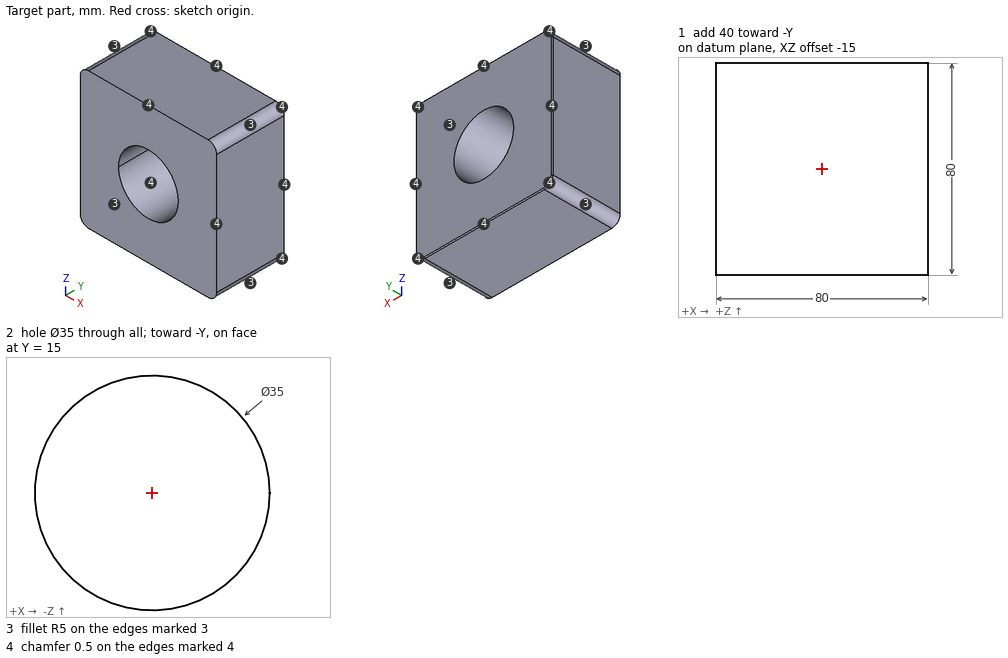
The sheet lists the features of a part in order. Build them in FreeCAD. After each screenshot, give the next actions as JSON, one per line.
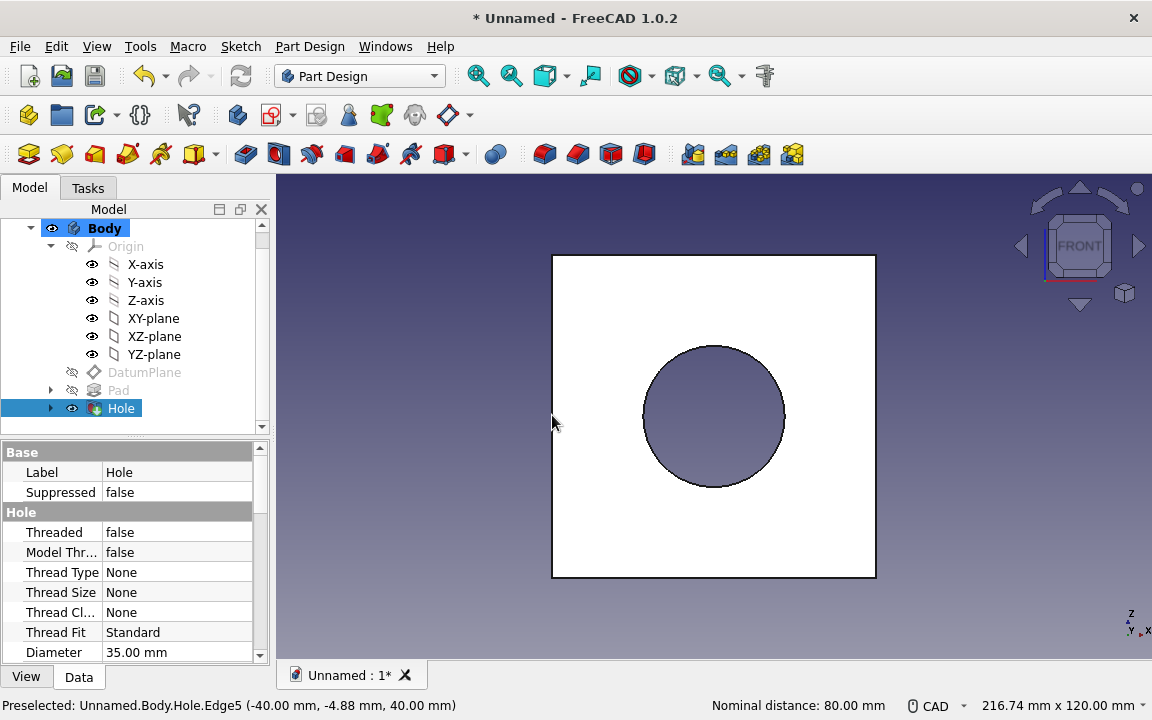
{"action": "key", "text": "3"}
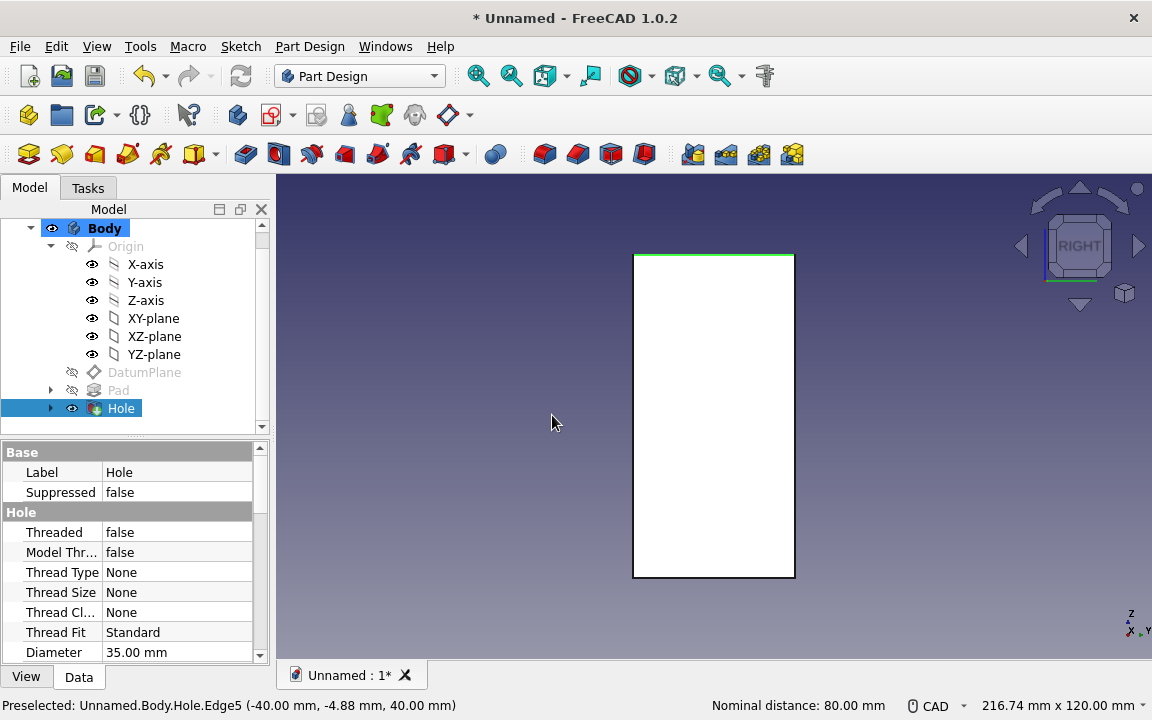
{"action": "left_click", "coordinate": [714, 577], "text": "ctrl"}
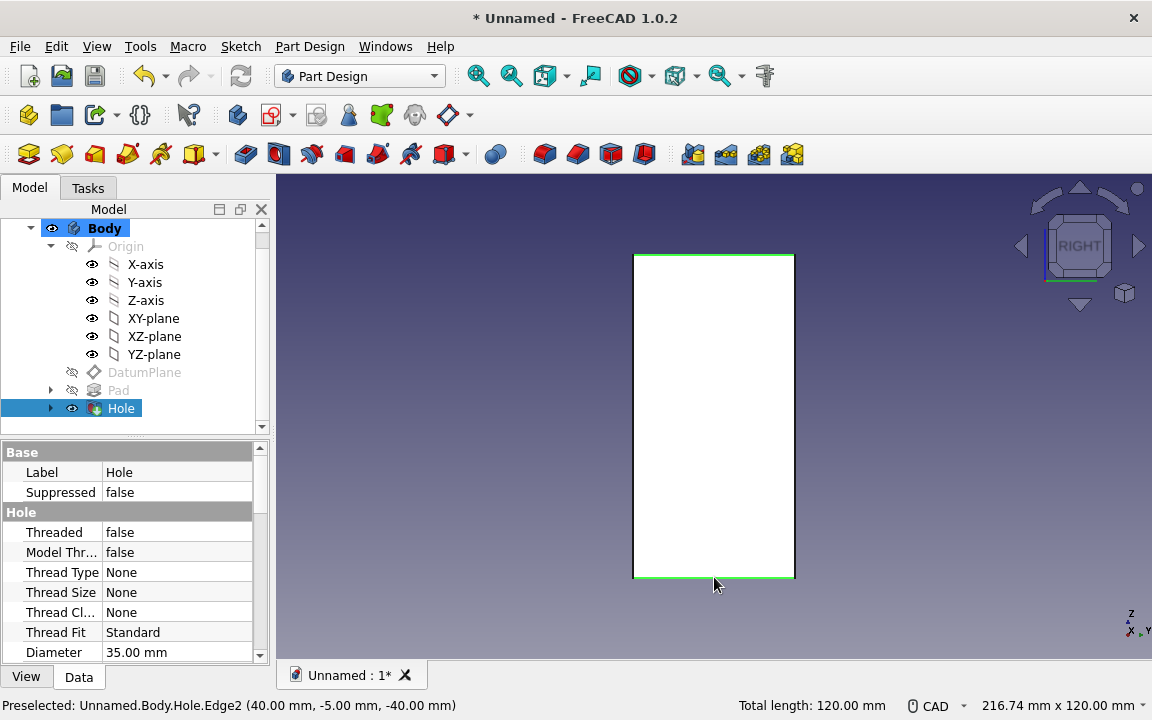
{"action": "key", "text": "5"}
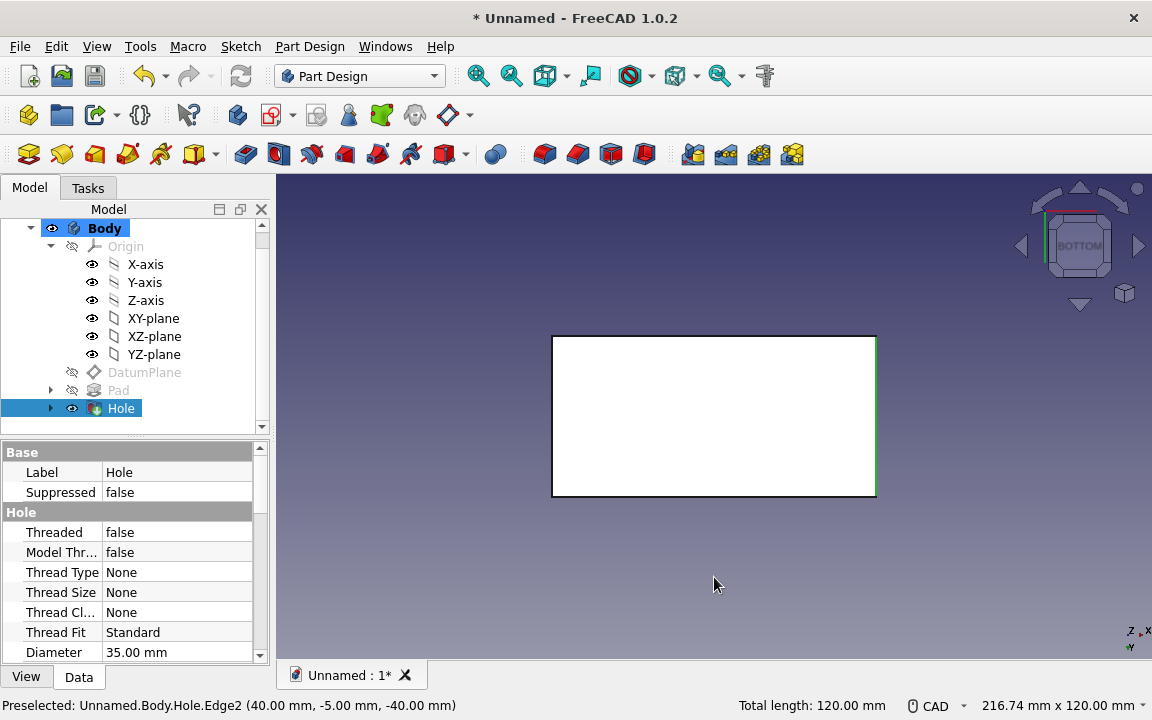
{"action": "left_click", "coordinate": [479, 76]}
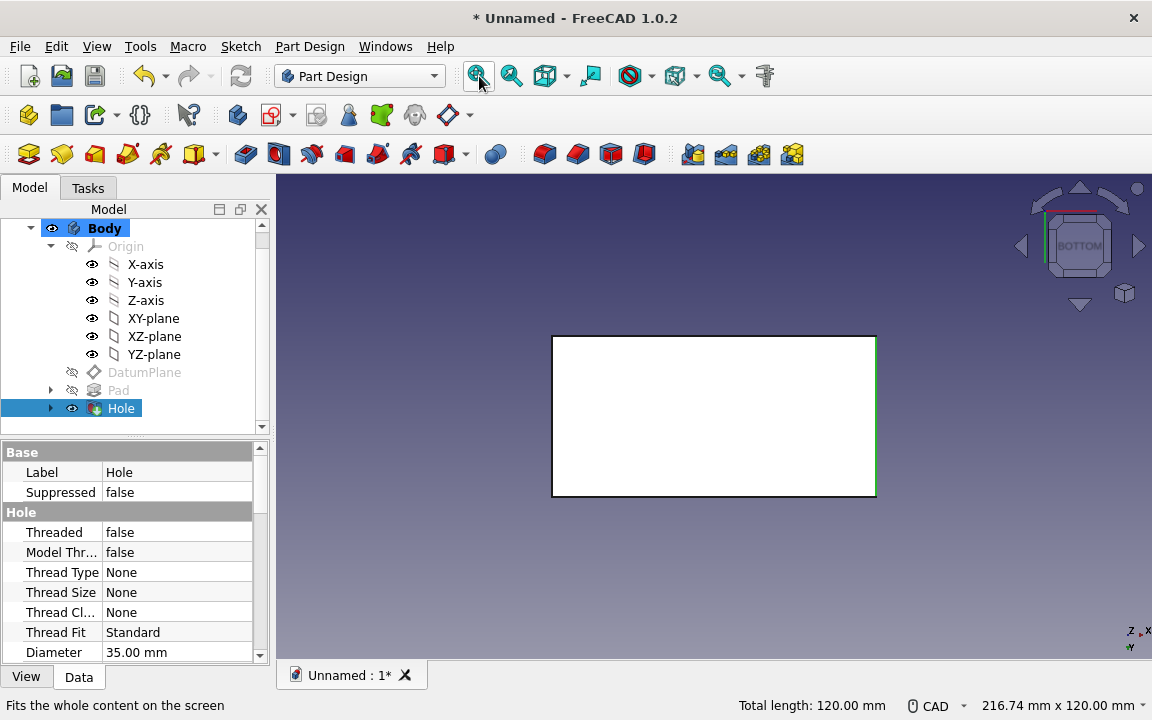
{"action": "left_click", "coordinate": [552, 415], "text": "ctrl"}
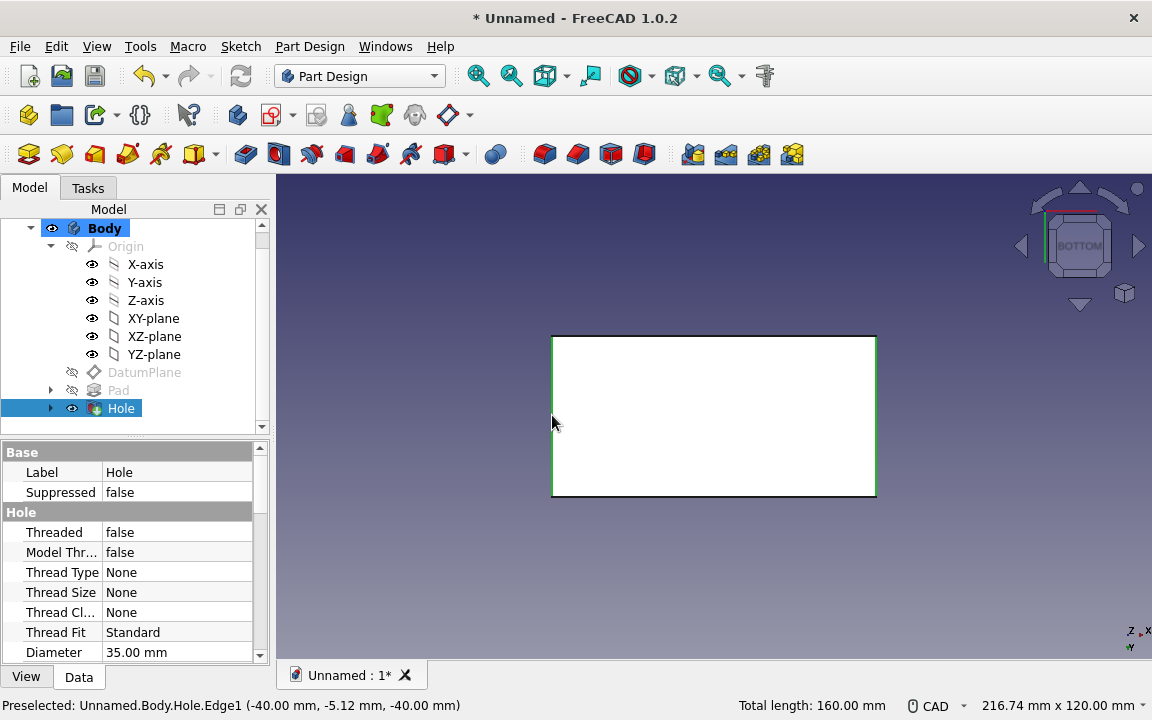
{"action": "left_click", "coordinate": [545, 154]}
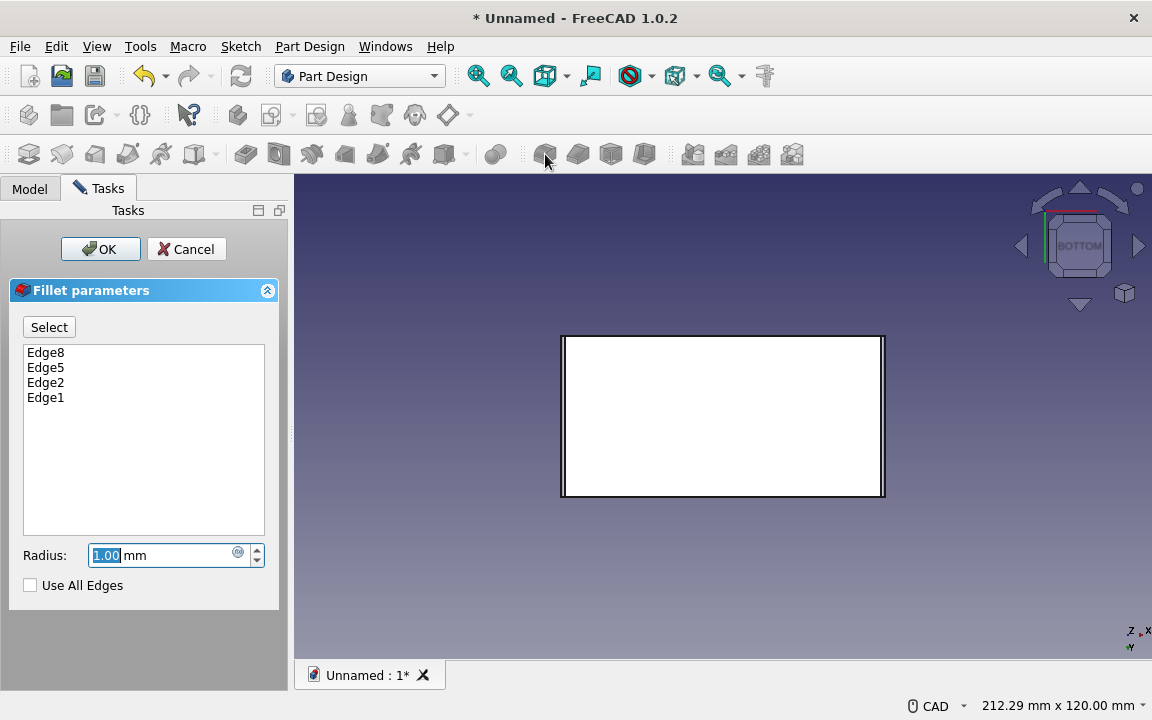
{"action": "type", "text": "5"}
{"action": "key", "text": "Tab"}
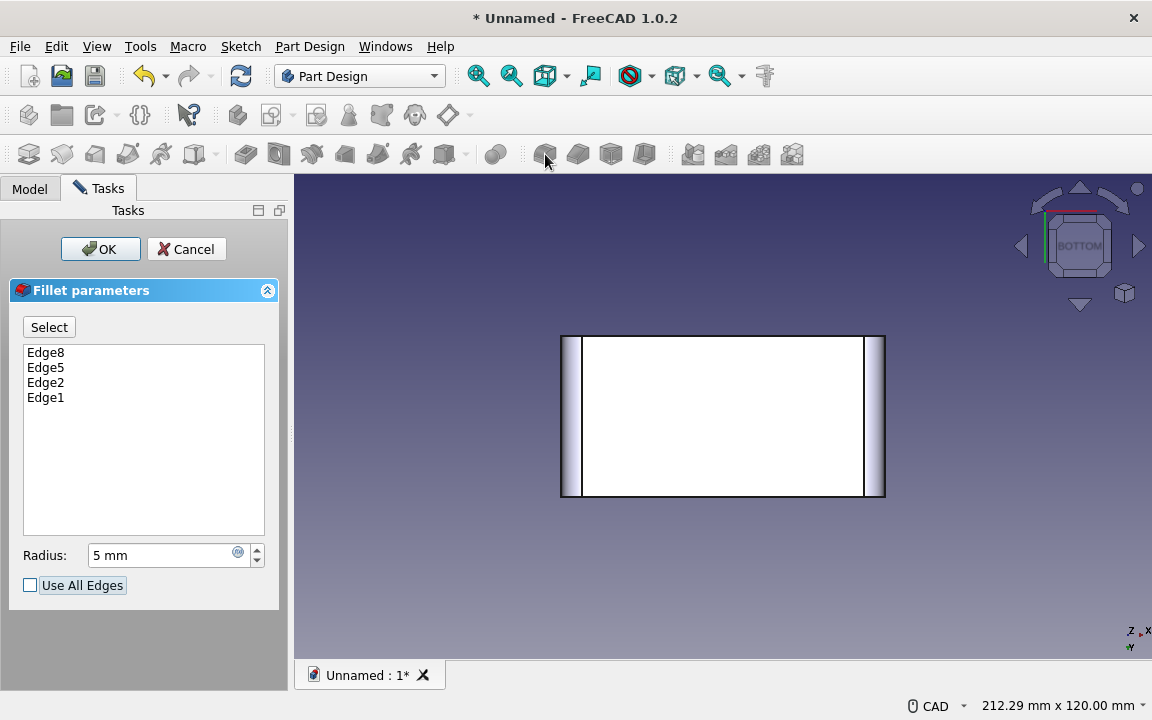
{"action": "left_click", "coordinate": [101, 249]}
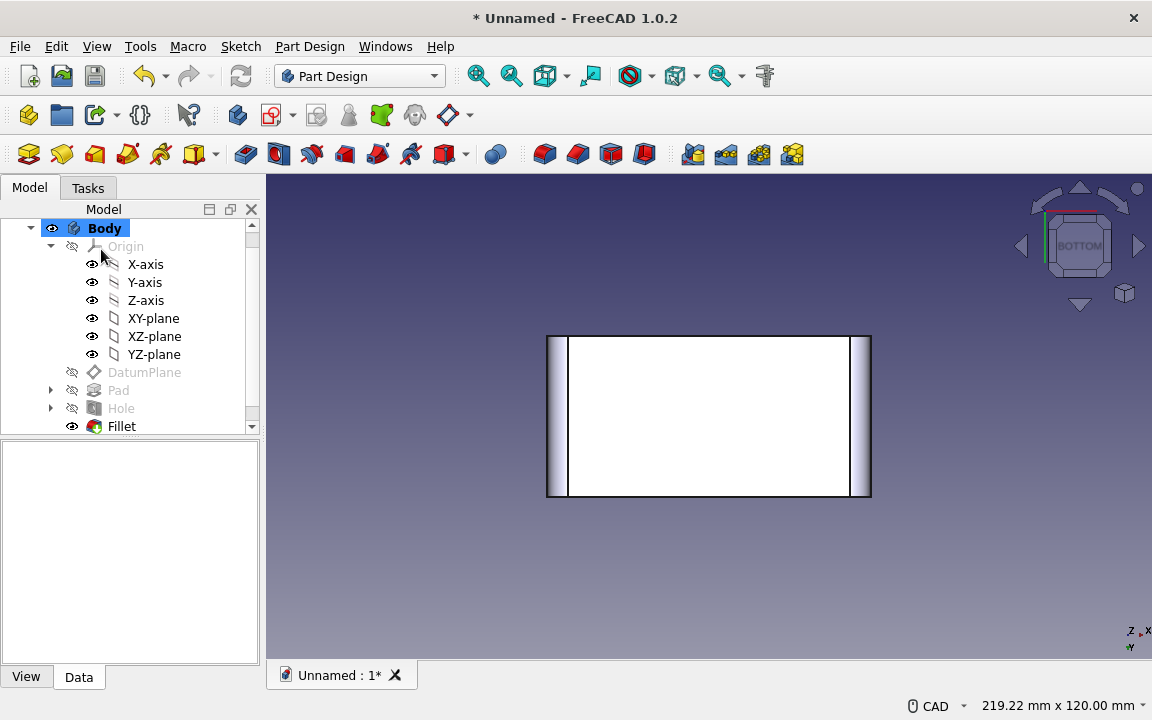
{"action": "left_click", "coordinate": [479, 76]}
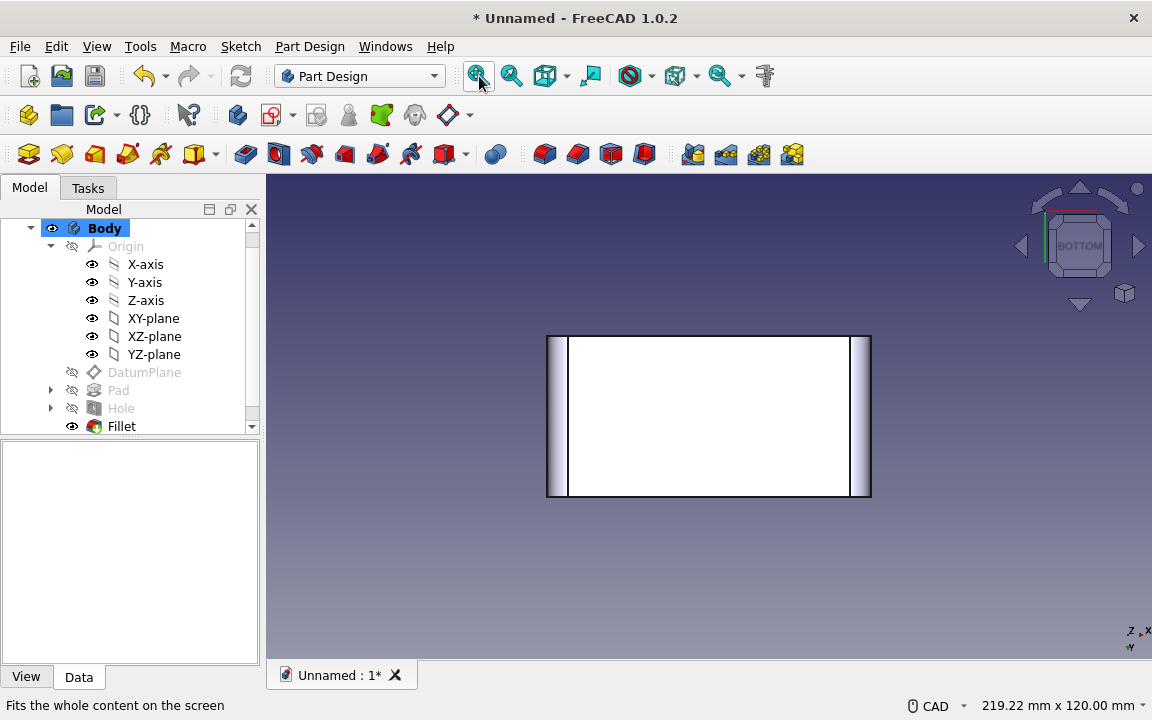
{"action": "left_click", "coordinate": [553, 496]}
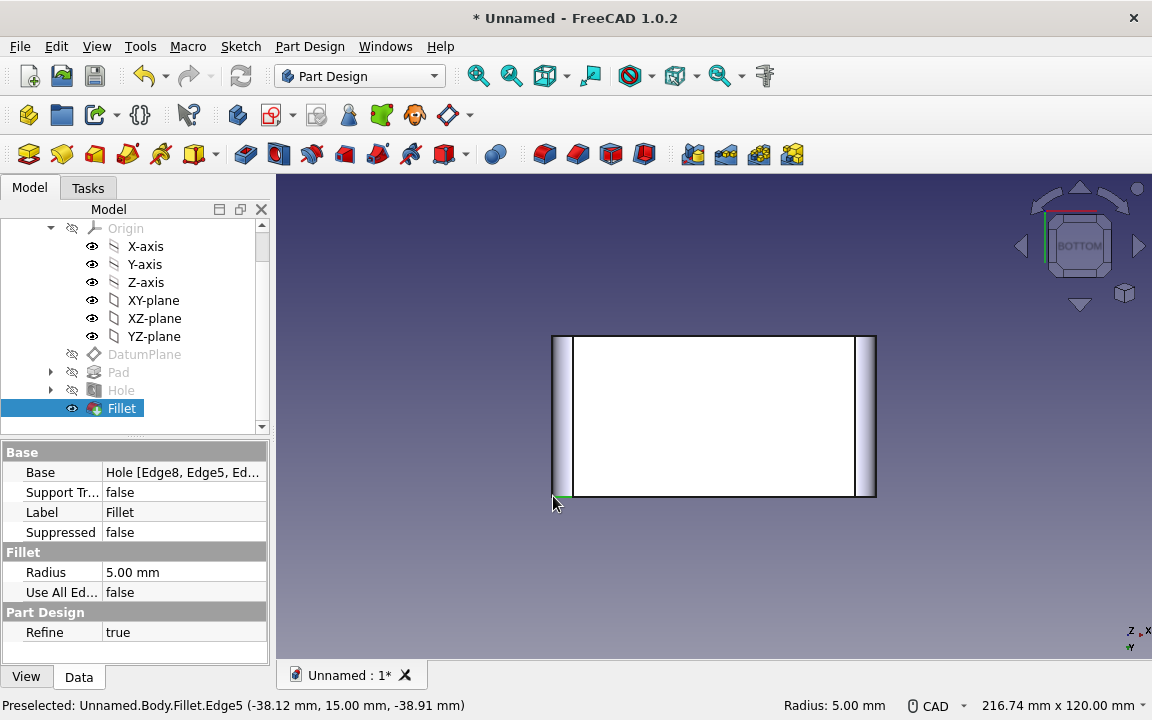
{"action": "left_click", "coordinate": [870, 496], "text": "ctrl"}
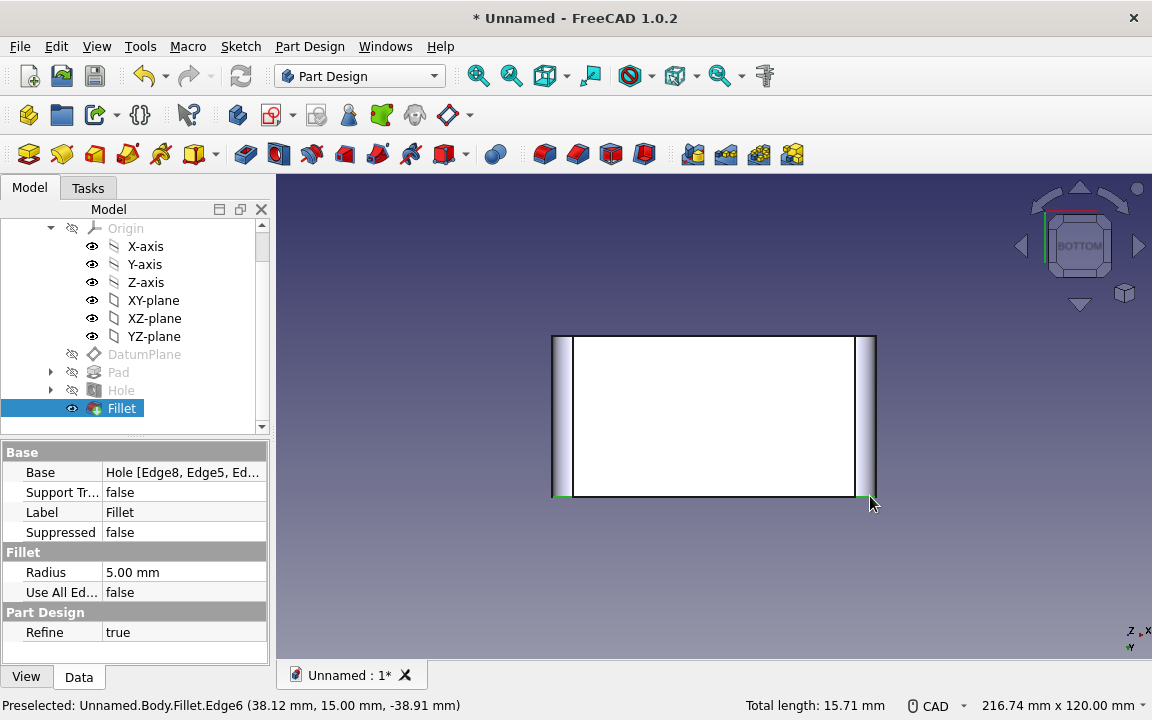
{"action": "key", "text": "0"}